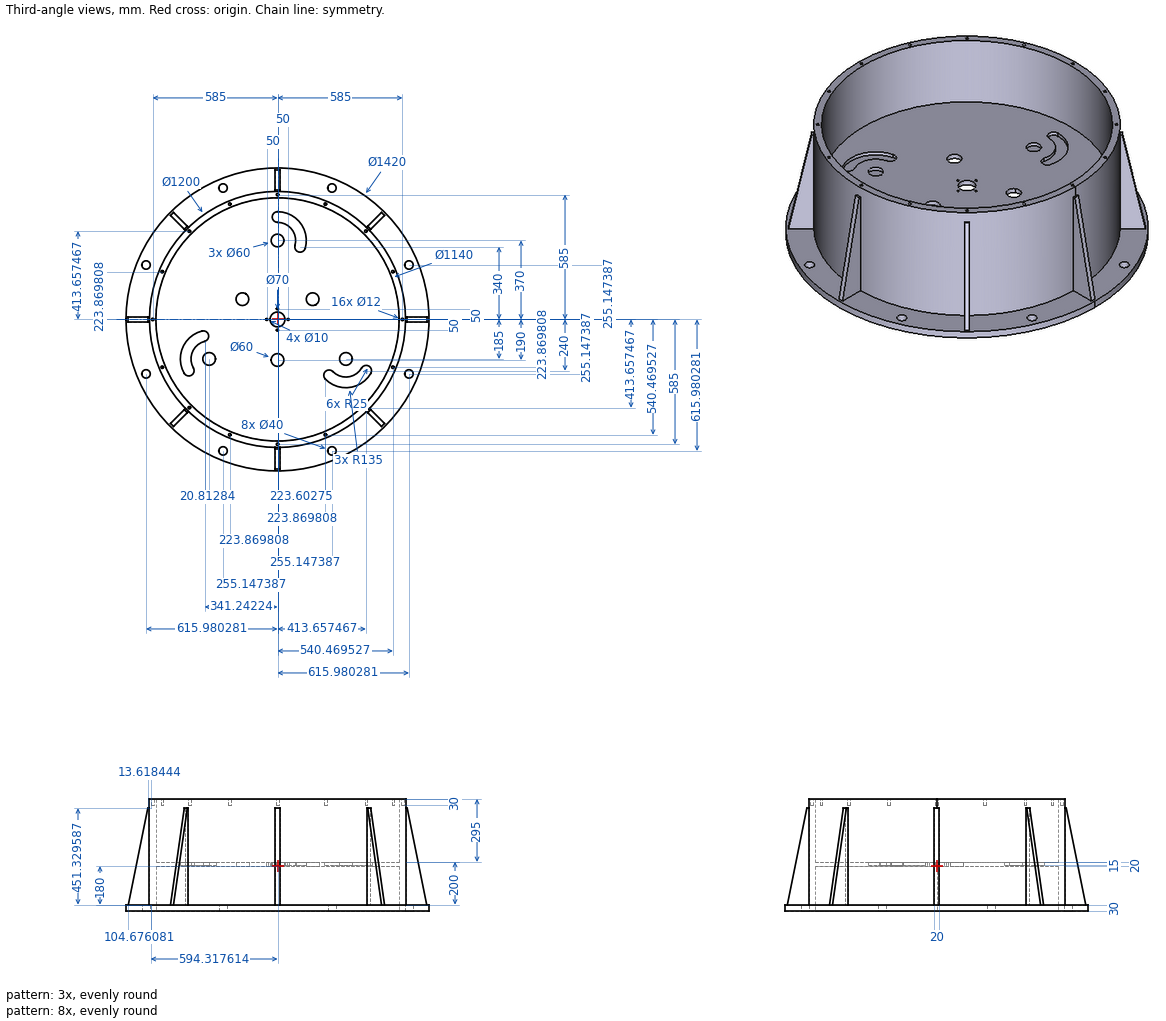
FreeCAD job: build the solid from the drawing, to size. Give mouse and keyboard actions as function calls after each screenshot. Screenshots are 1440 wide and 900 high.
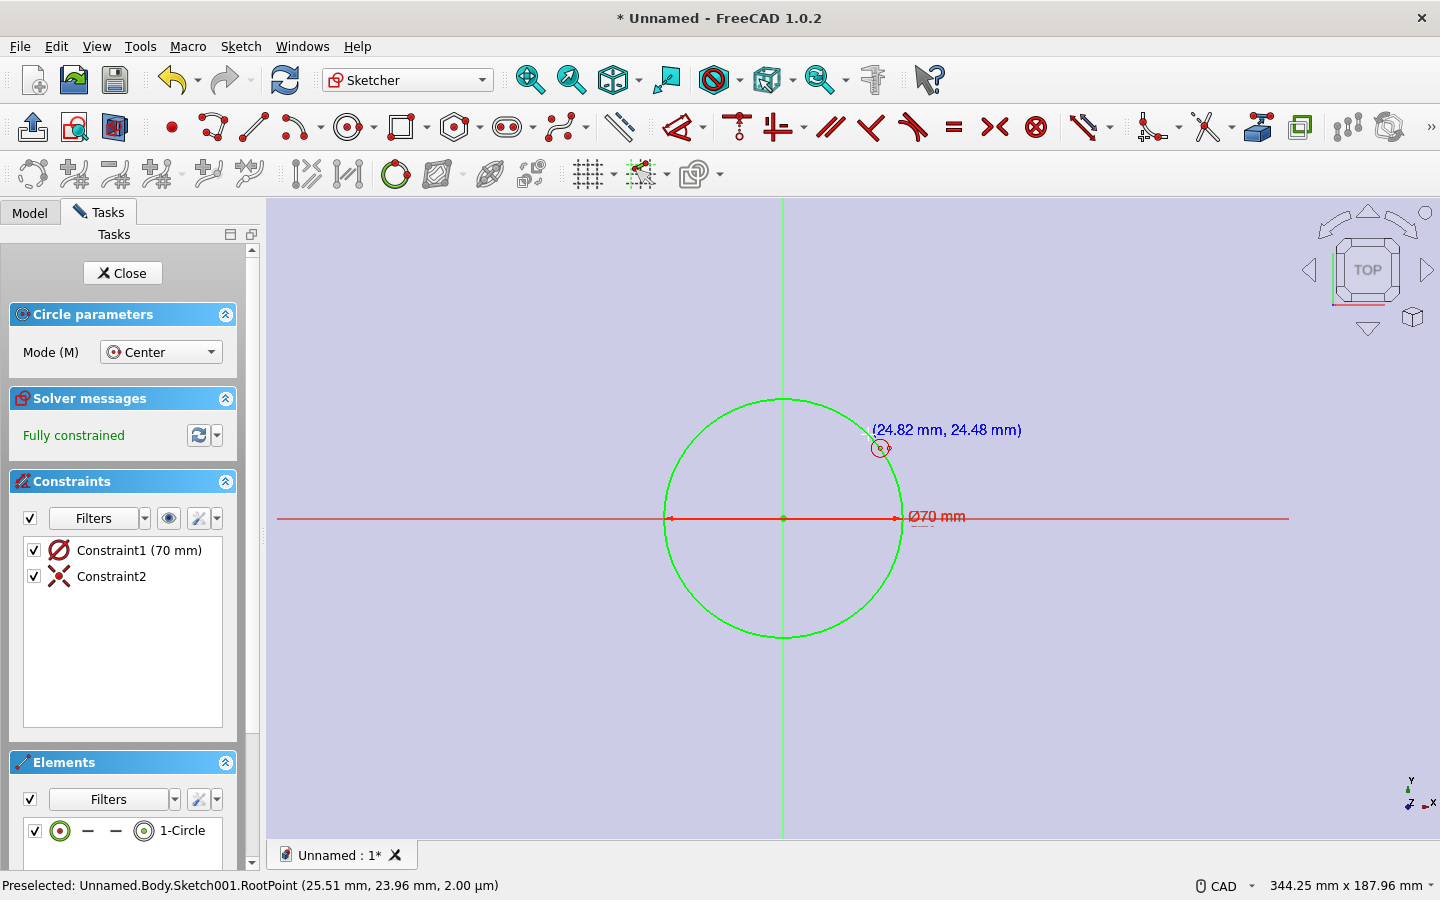
scroll(613, 518, up, 2)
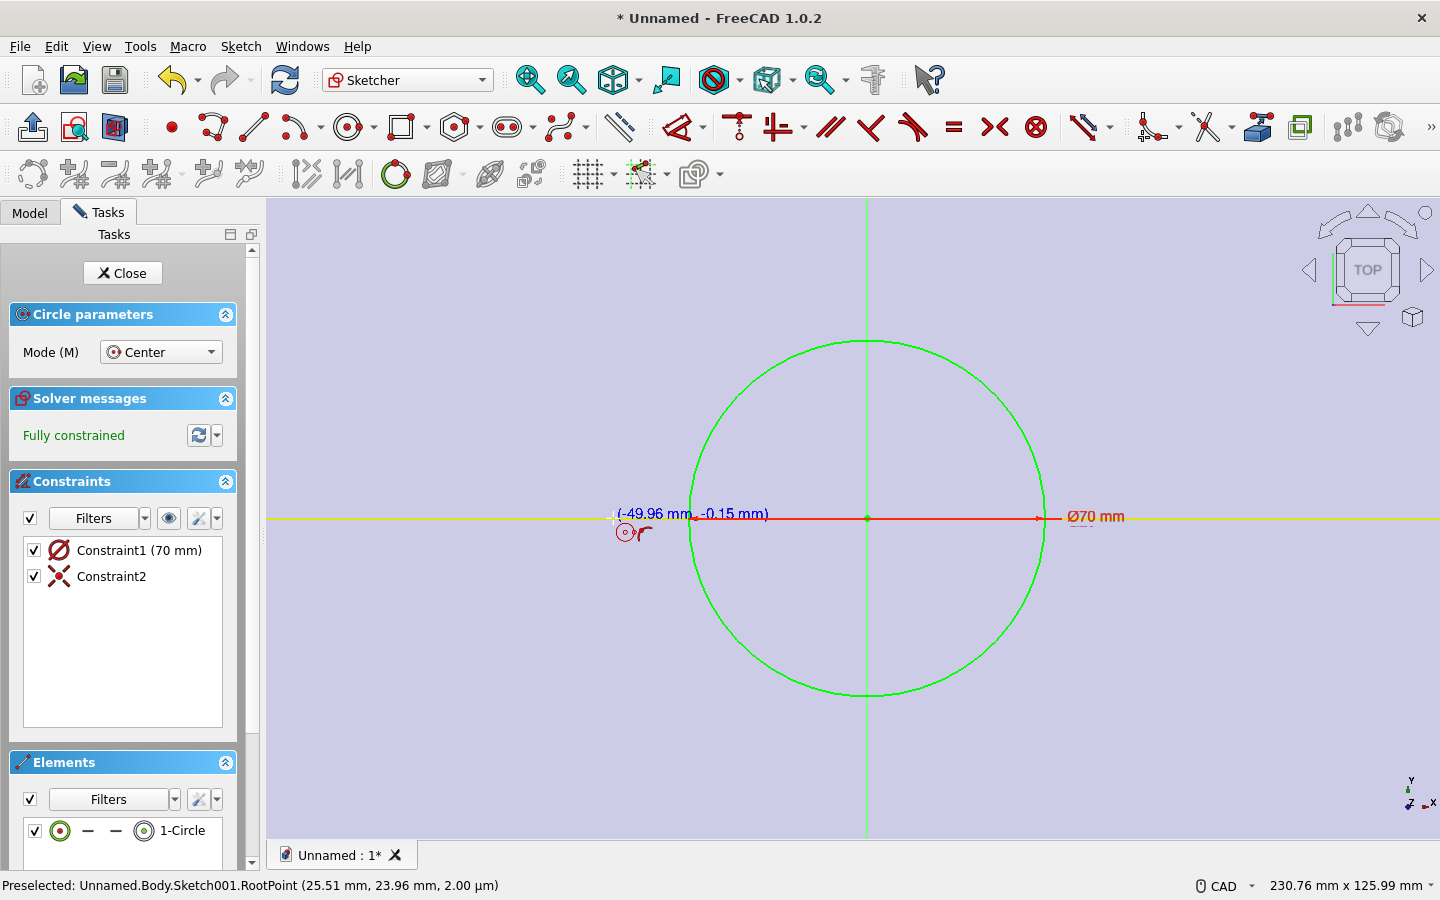
click(613, 518)
move(631, 501)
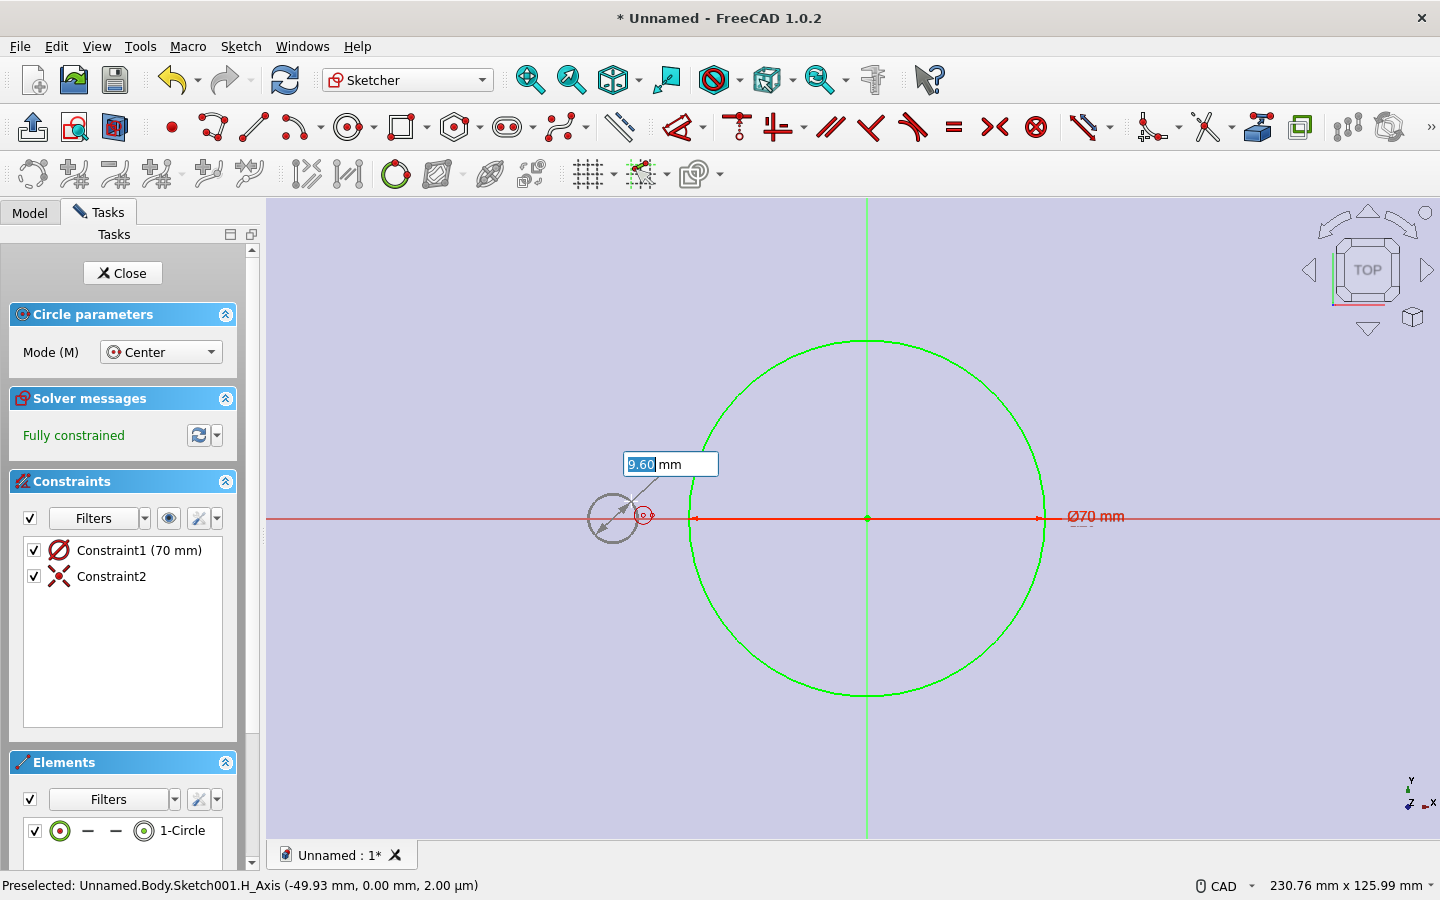
text(10)
key(Return)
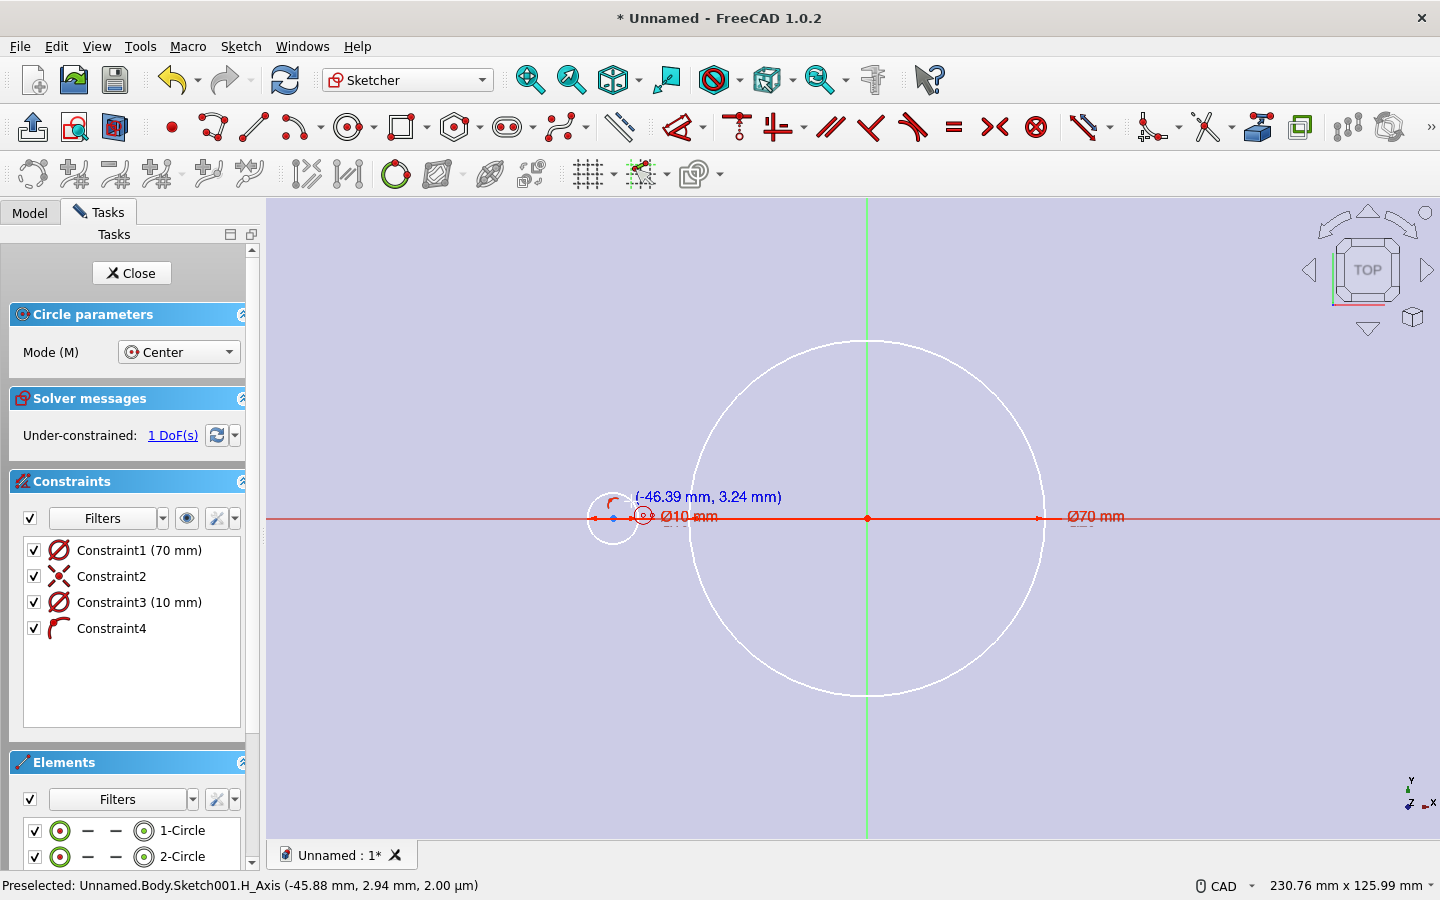
click(867, 773)
move(885, 755)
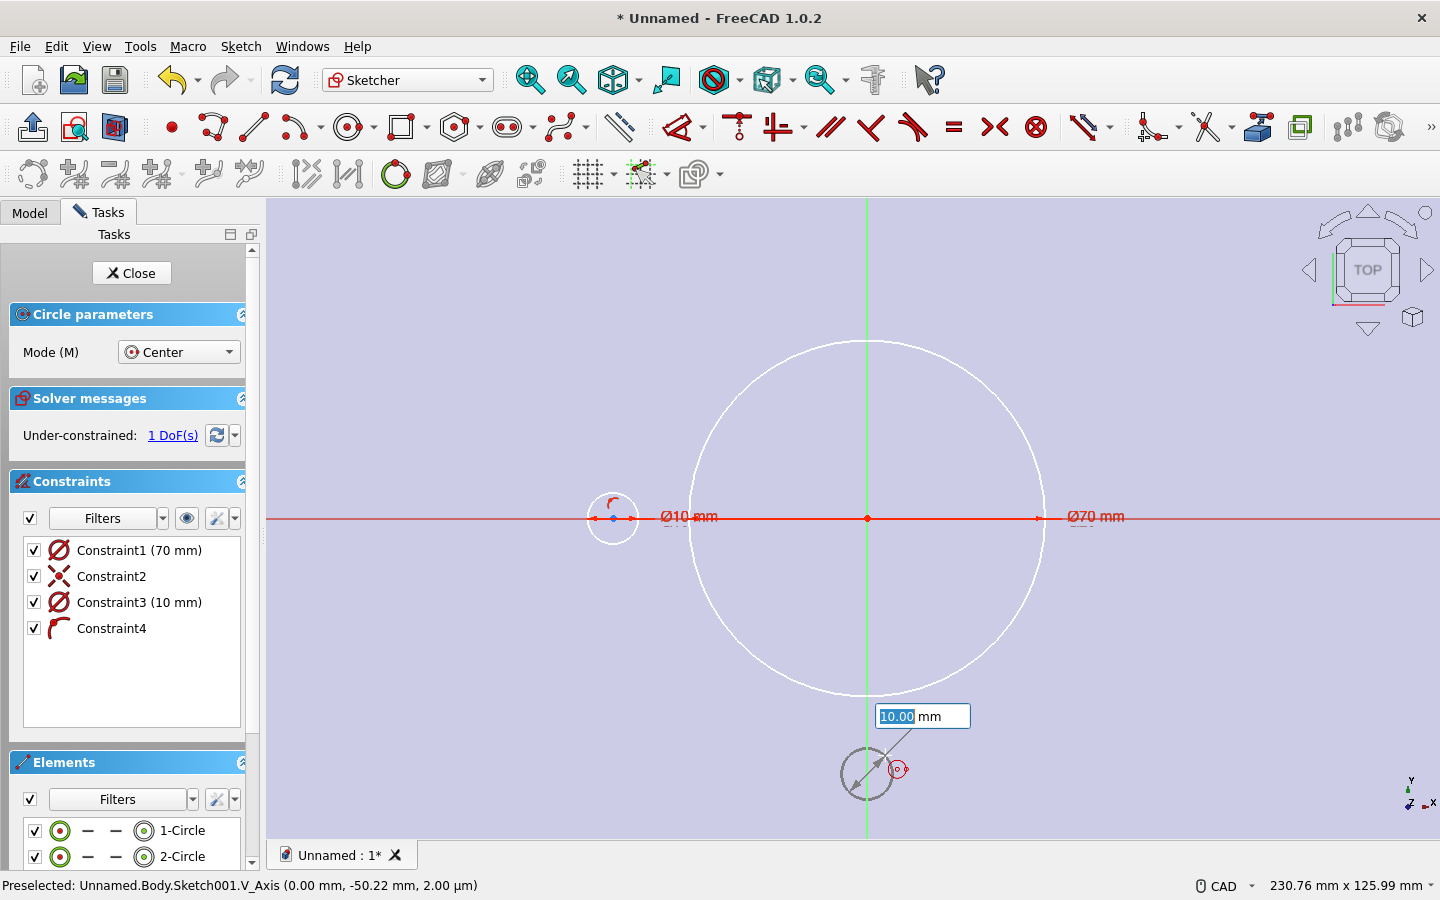
text(10)
key(Return)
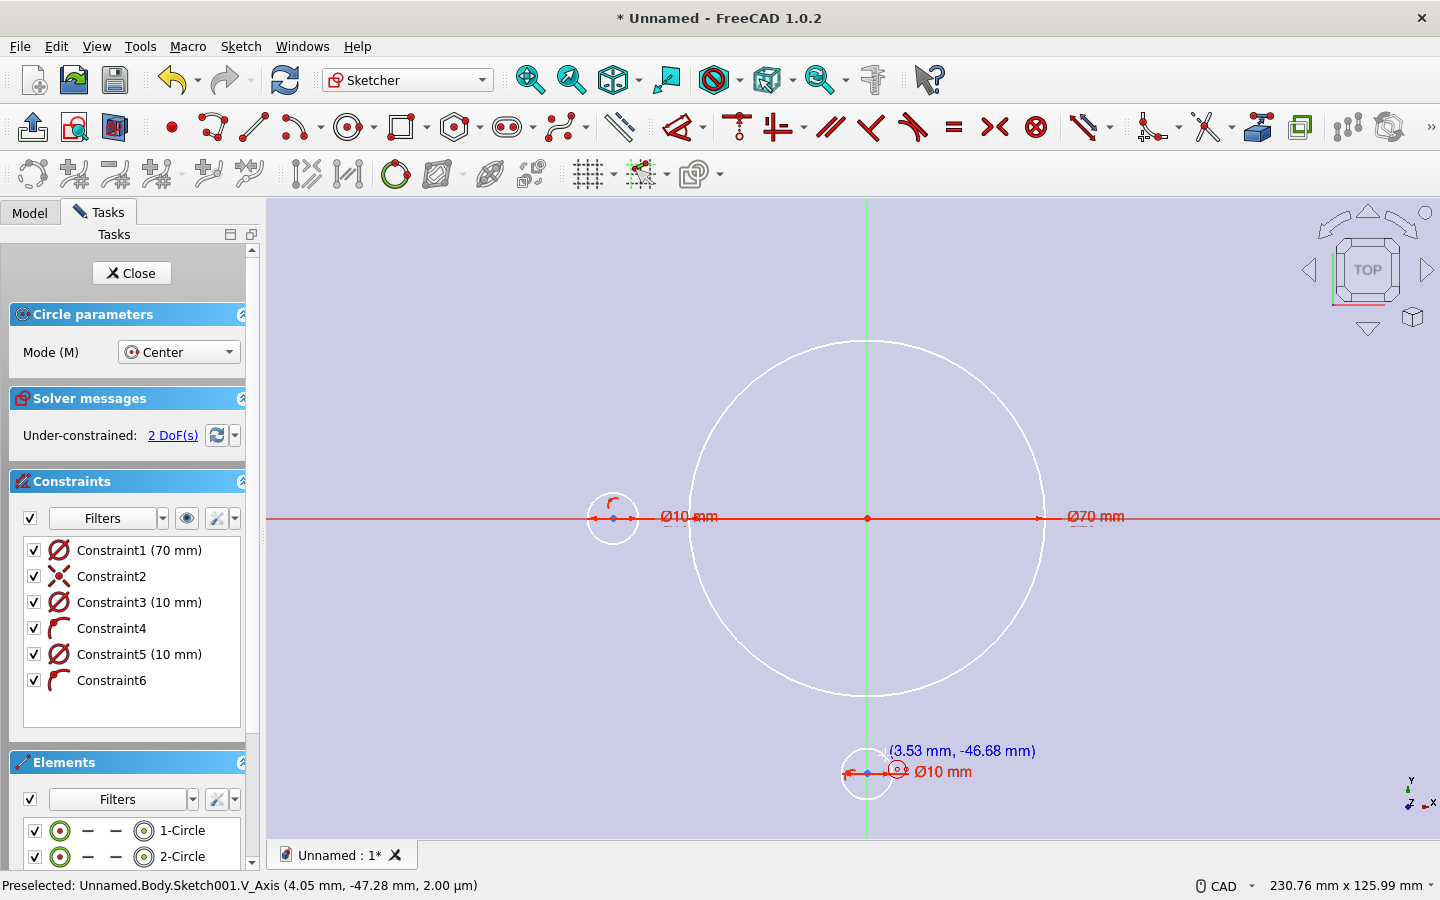
click(1121, 518)
move(1139, 501)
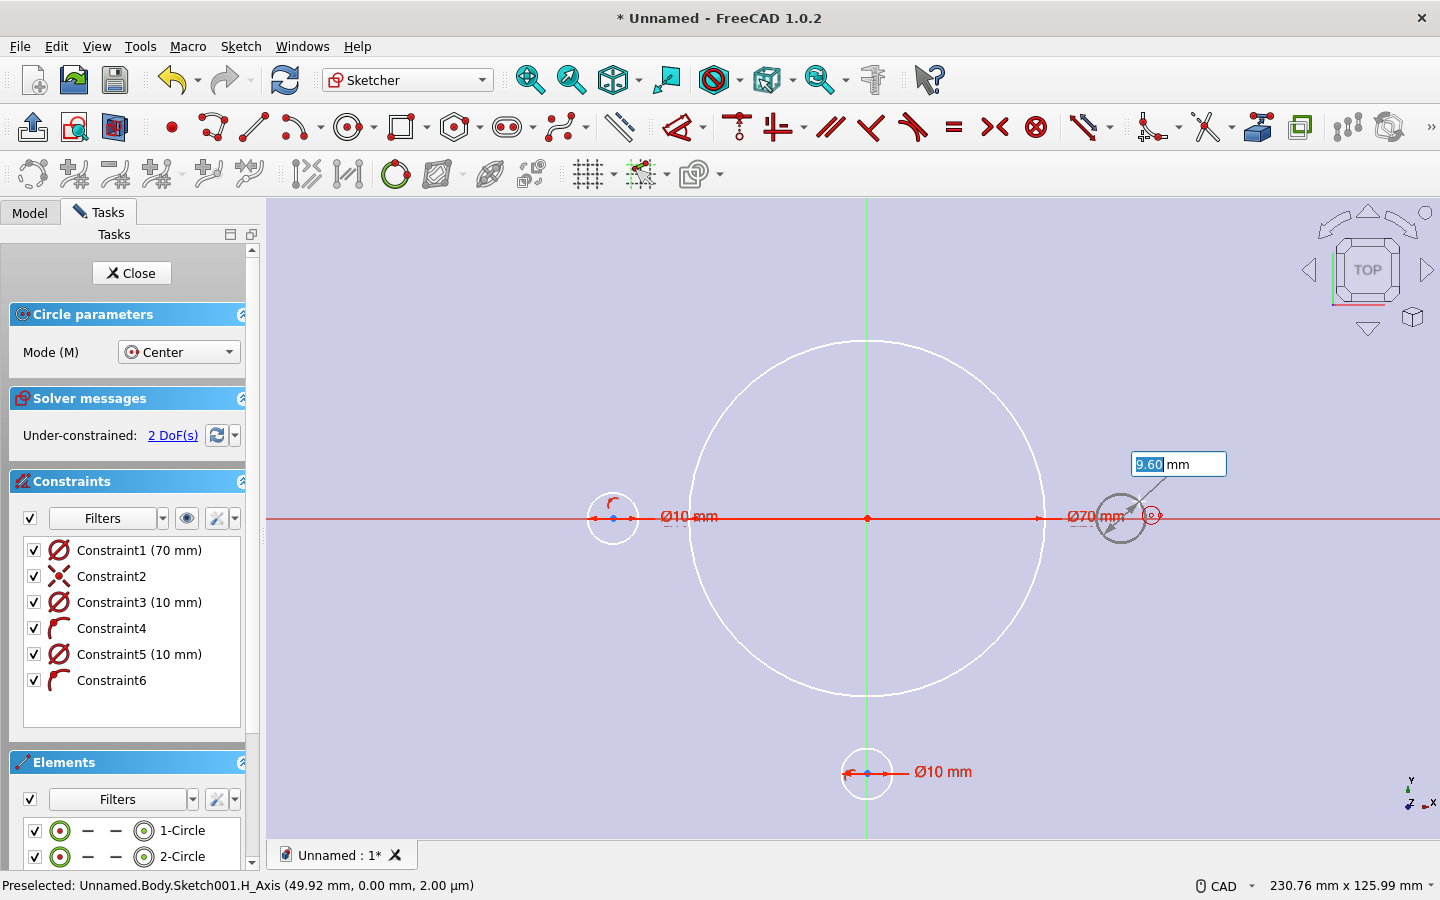
text(10)
key(Return)